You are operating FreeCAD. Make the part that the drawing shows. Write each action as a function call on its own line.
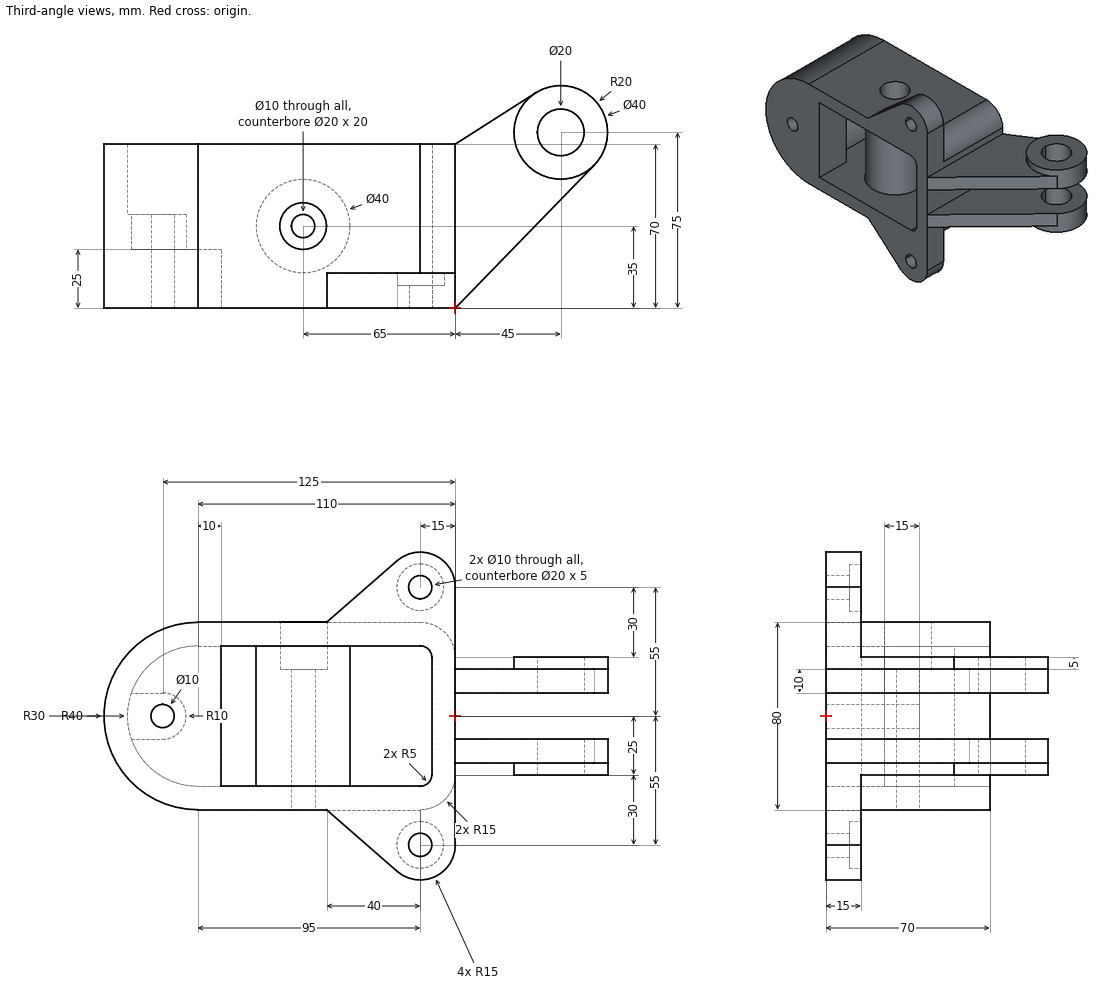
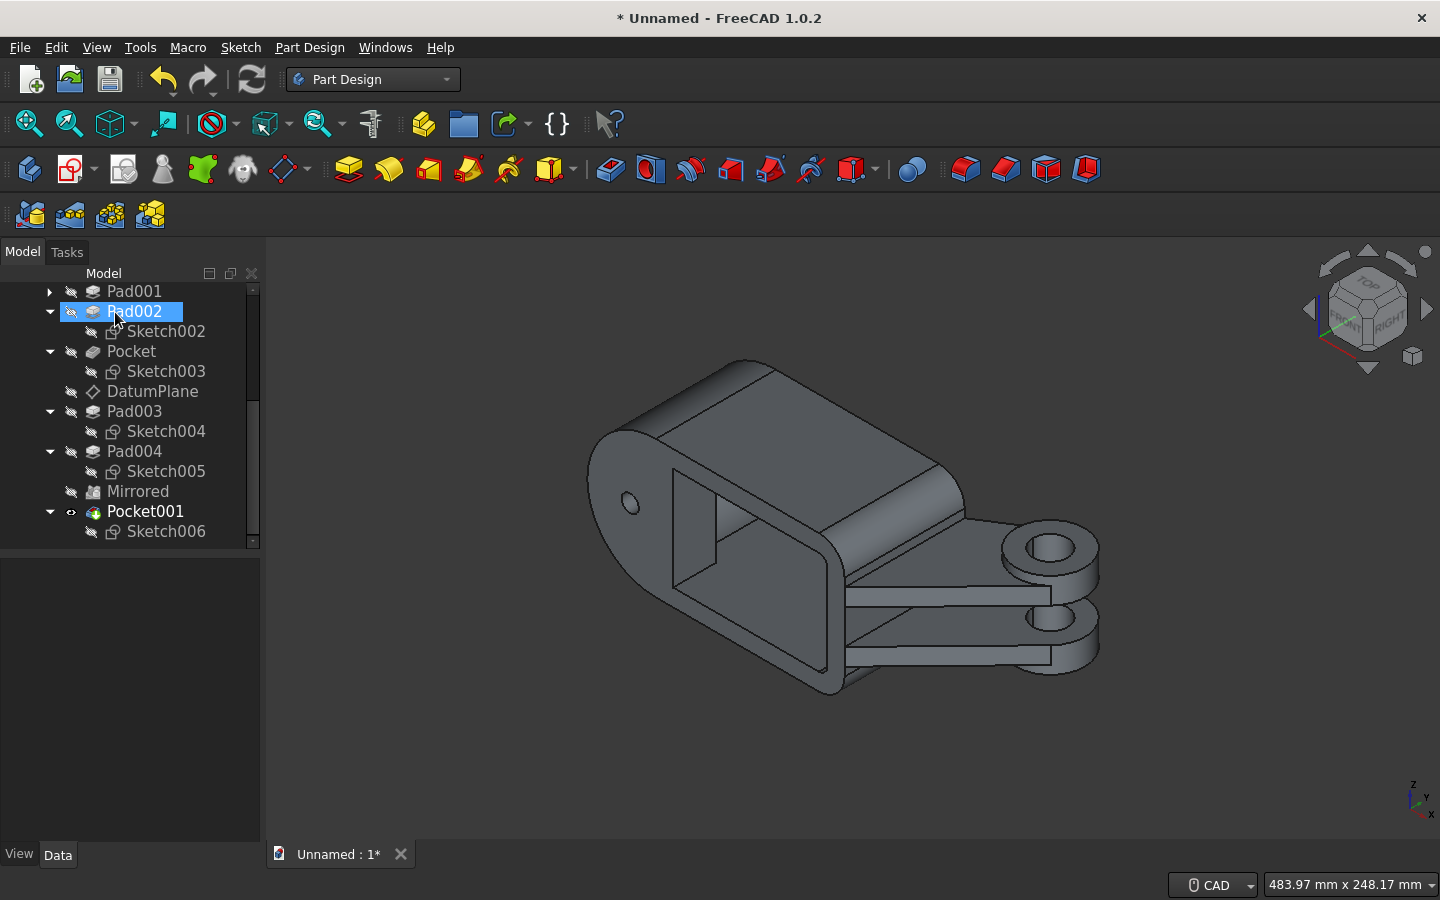
click(797, 450)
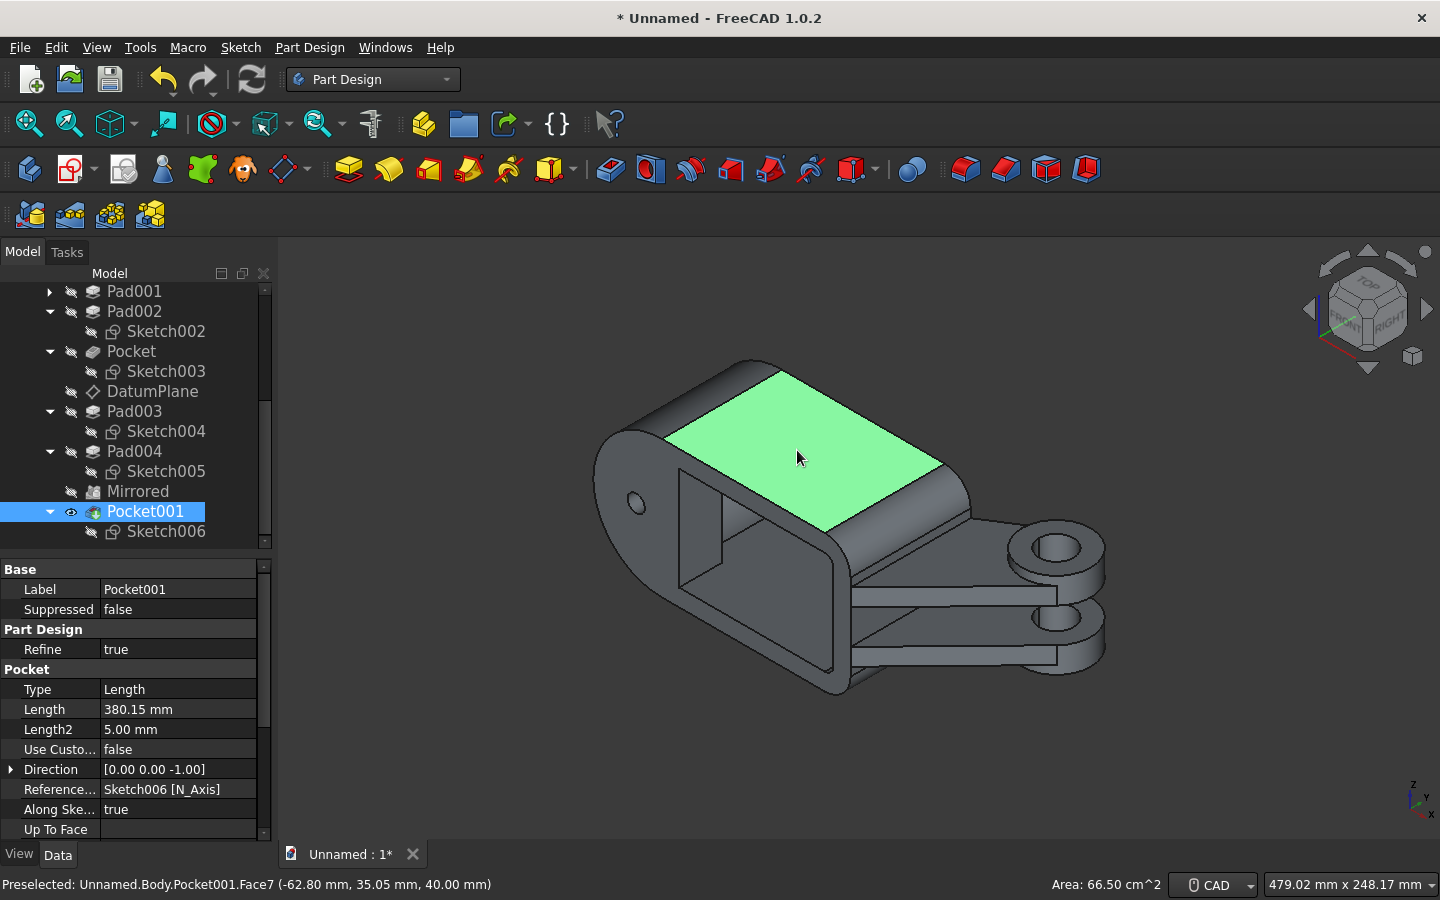
click(70, 170)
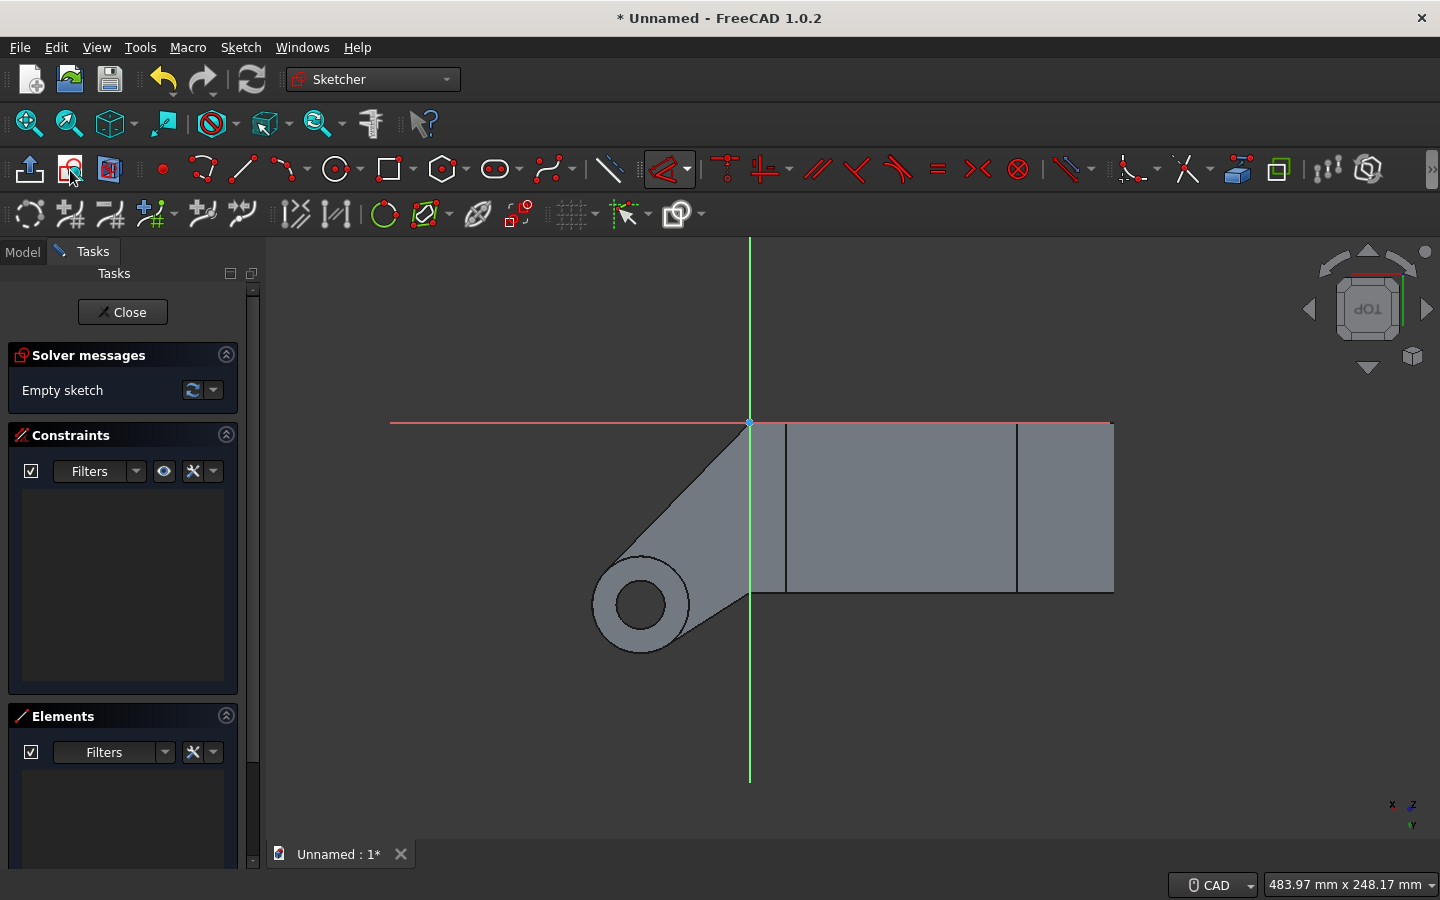
scroll(893, 461, up, 5)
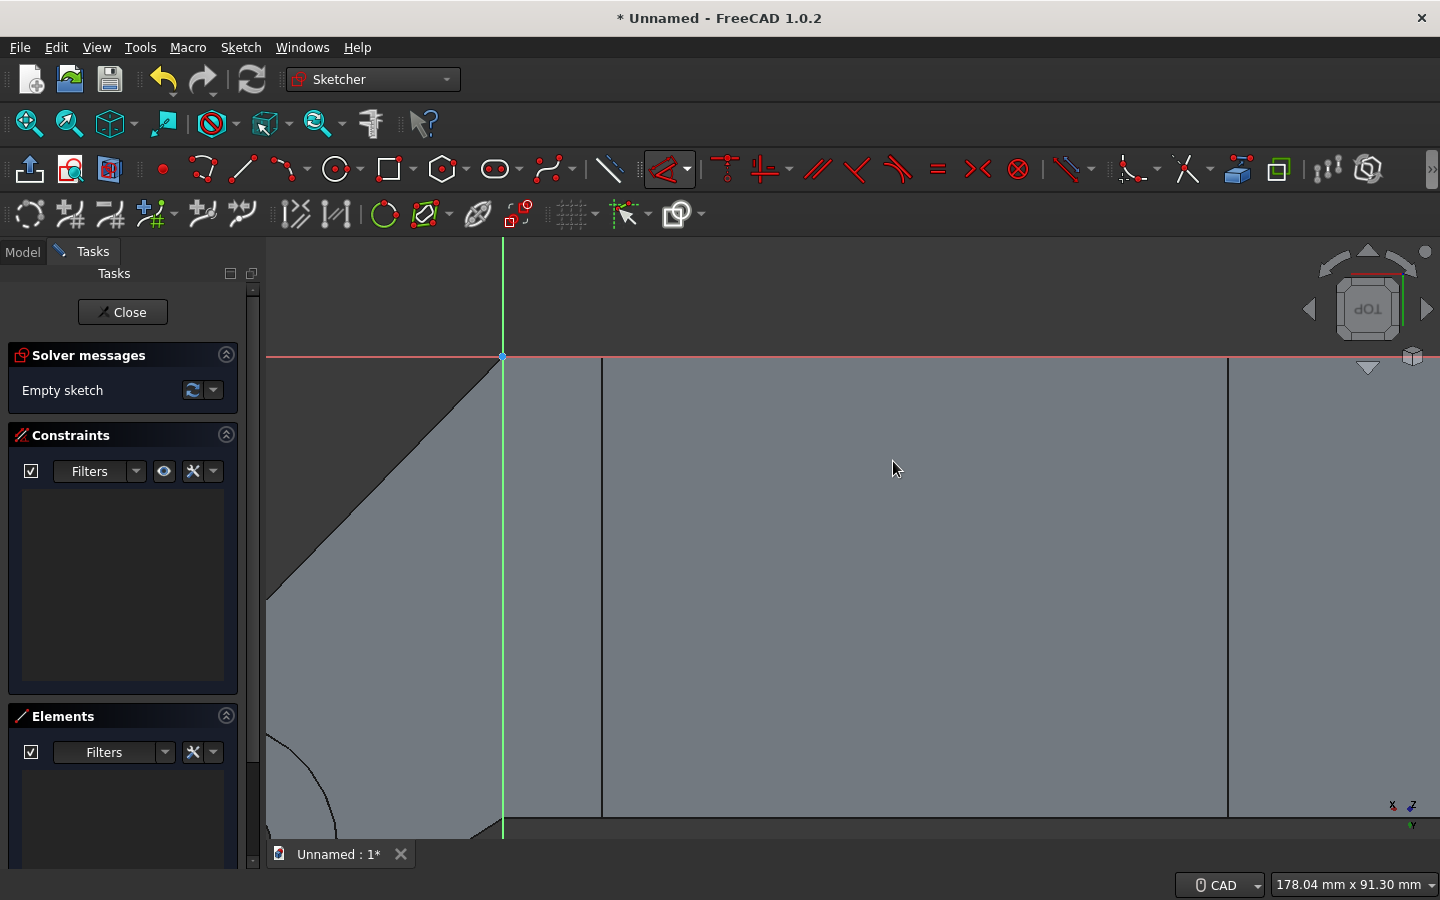
key(g)
key(c)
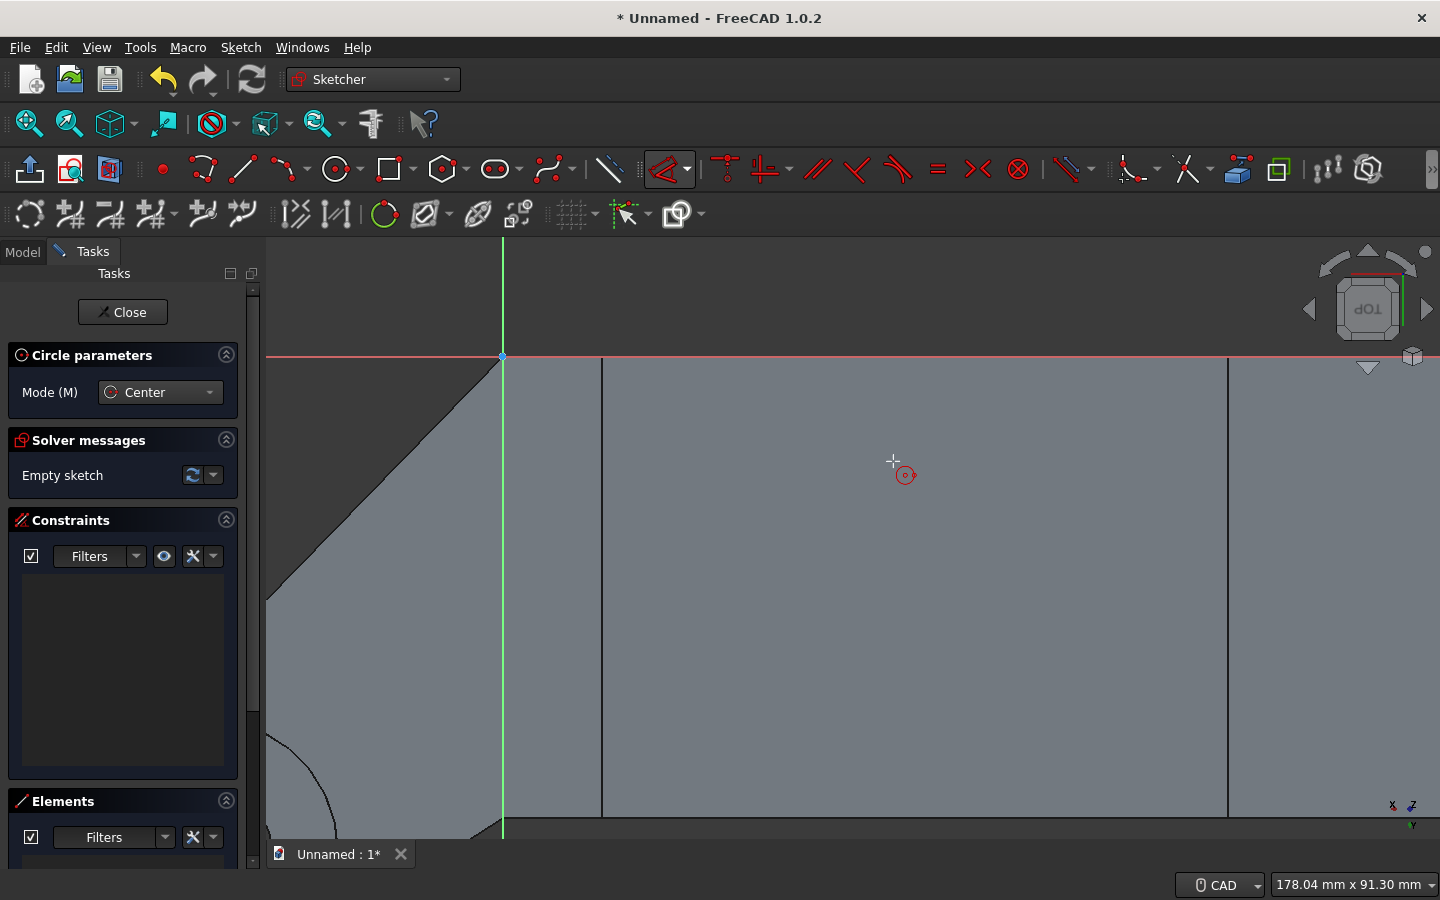
click(931, 588)
move(1025, 494)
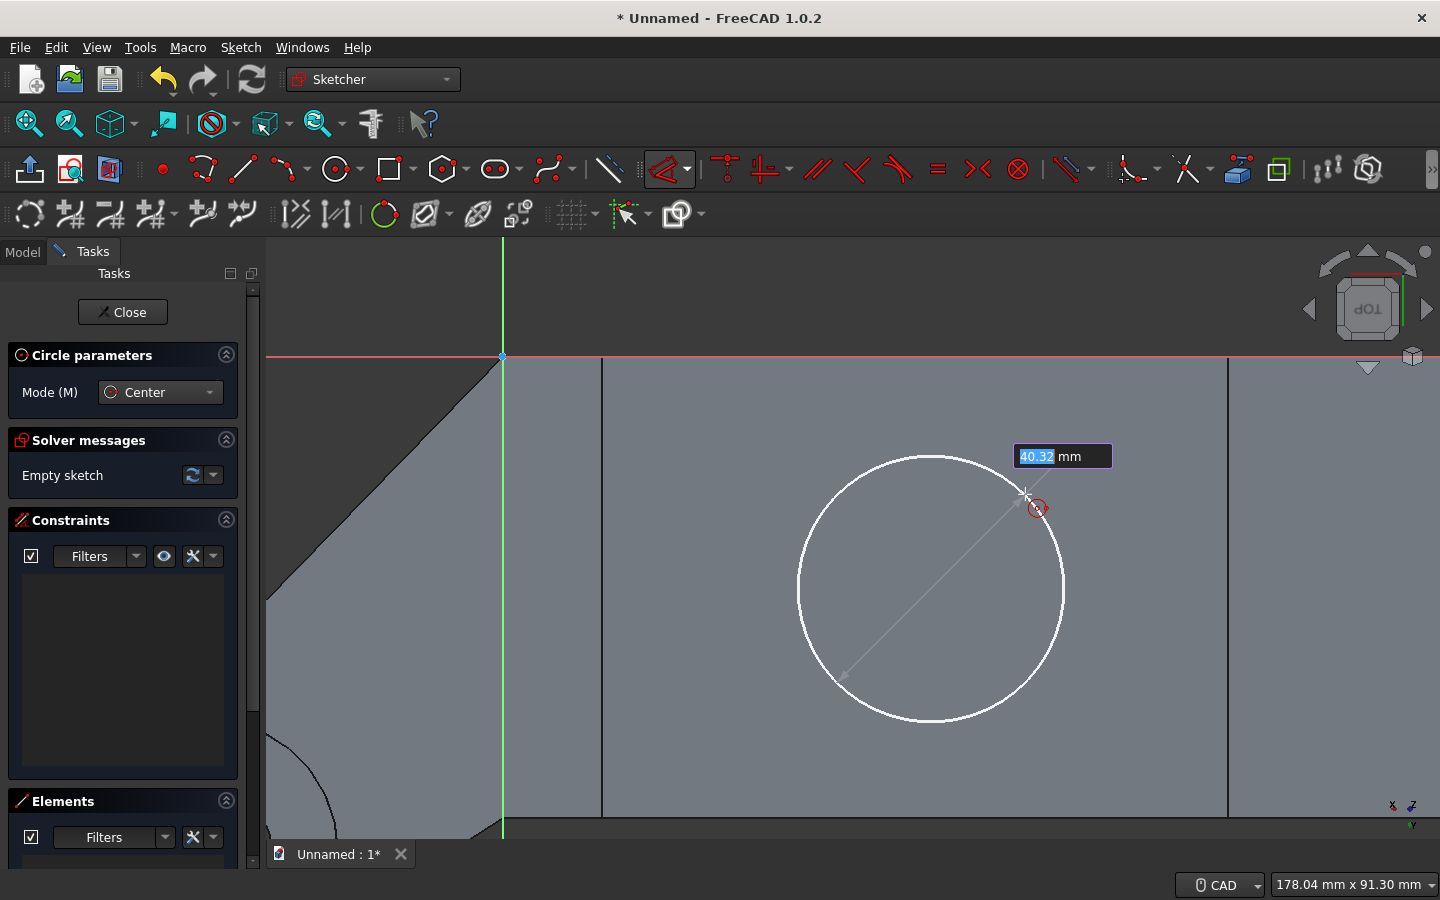
text(40)
key(Return)
key(Escape)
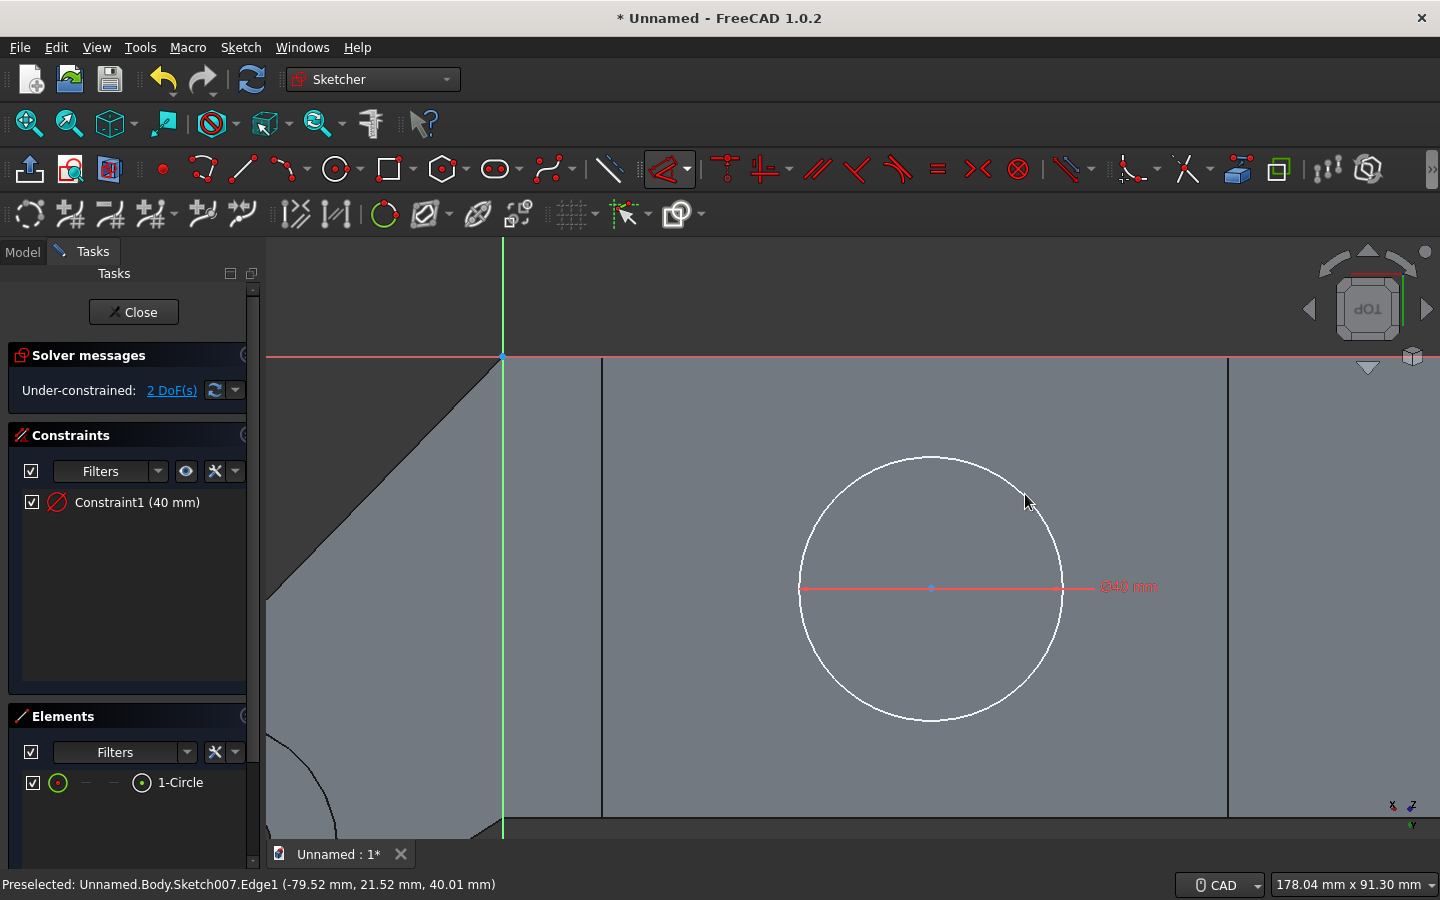
click(931, 589)